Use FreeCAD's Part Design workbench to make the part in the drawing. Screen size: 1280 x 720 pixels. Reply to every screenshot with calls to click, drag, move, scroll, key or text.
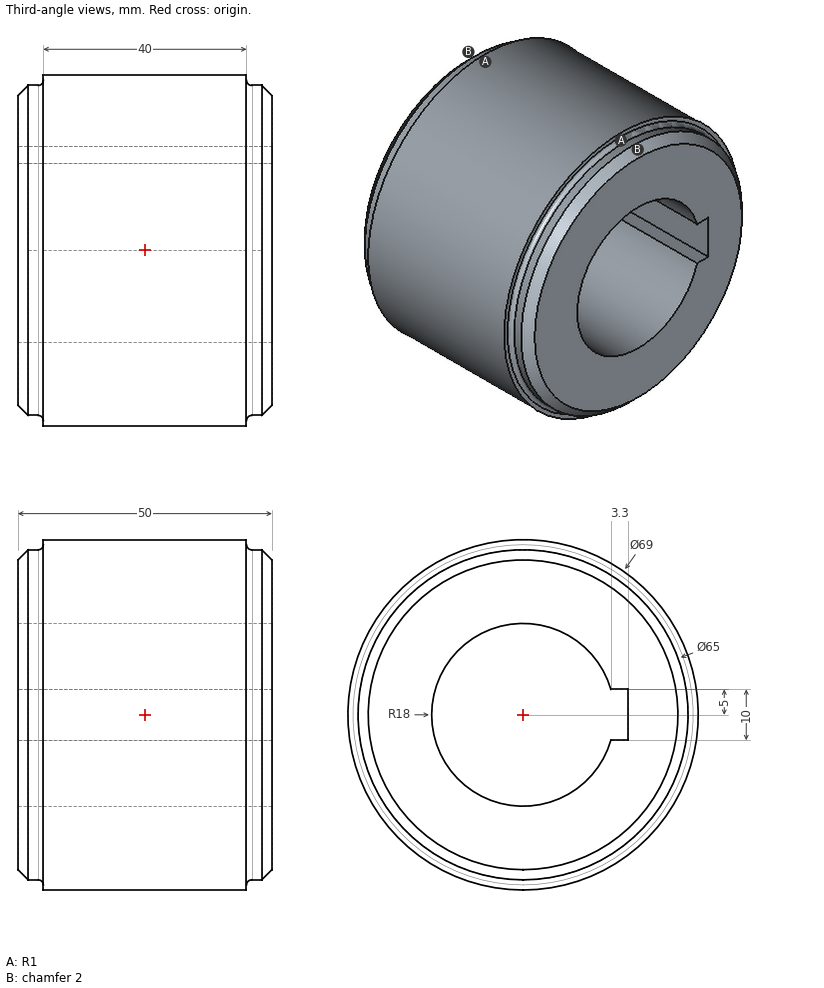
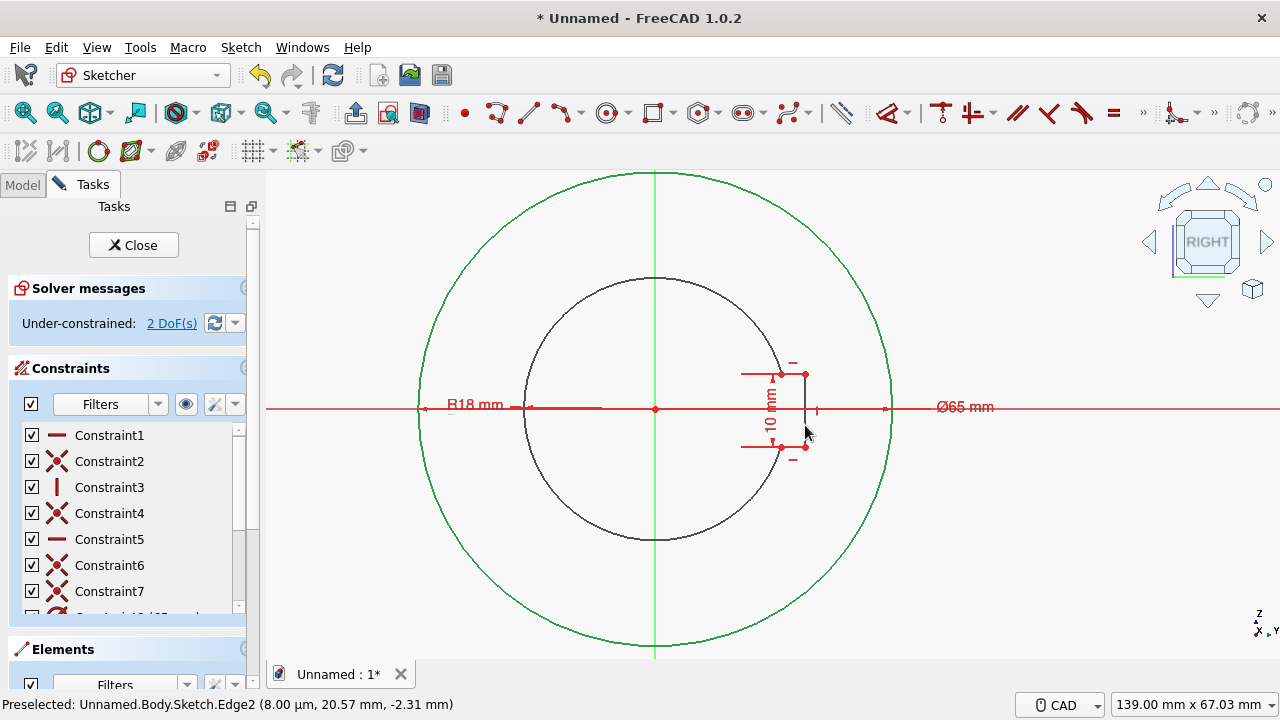
click(782, 374)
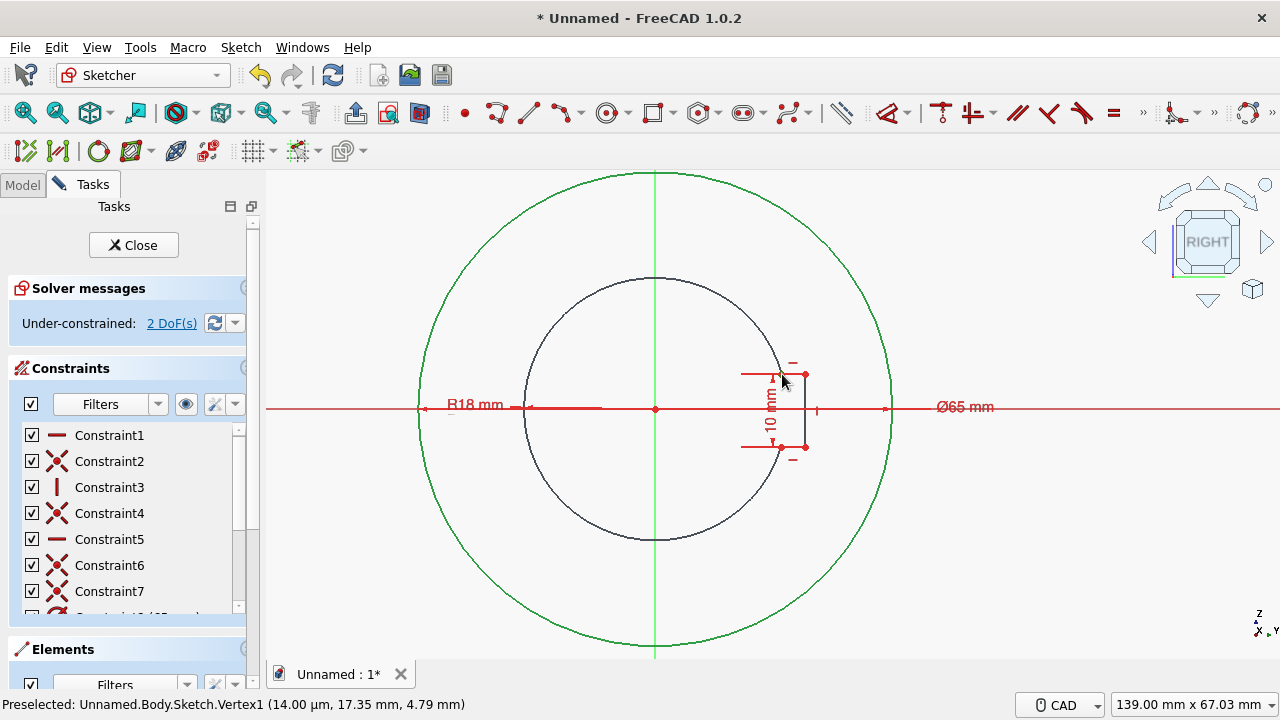
key(i)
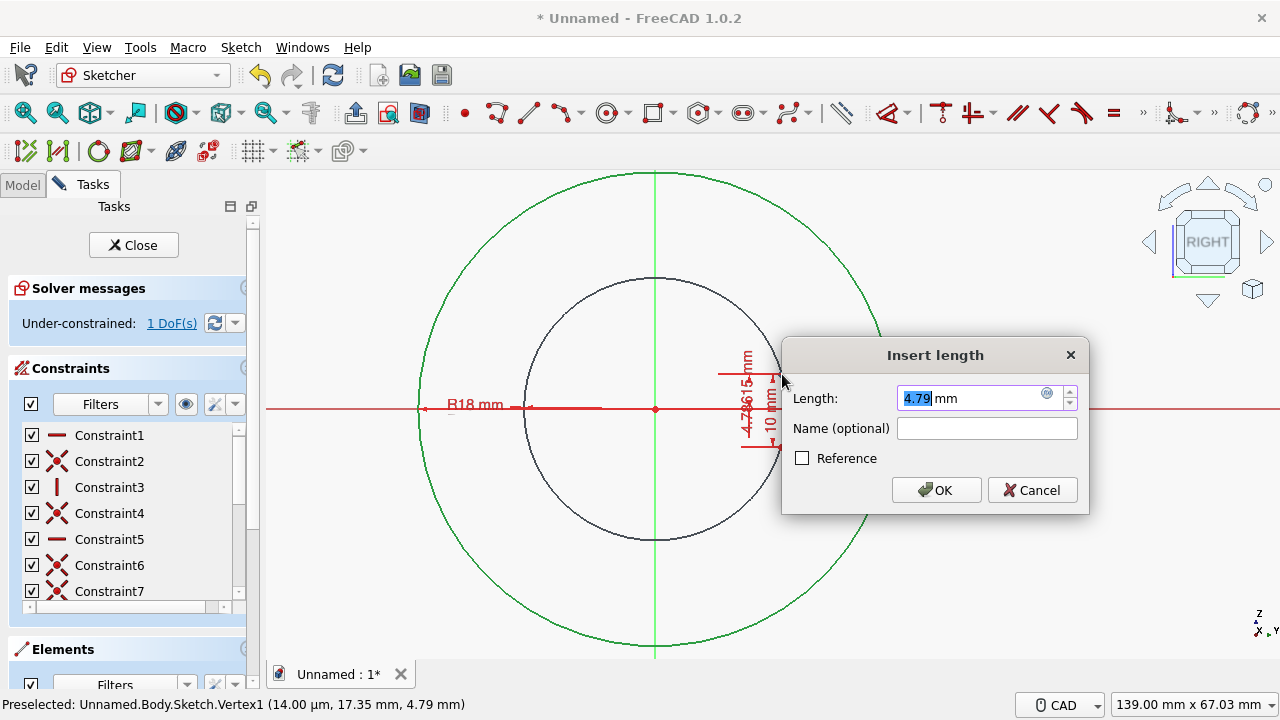
text(5)
key(Return)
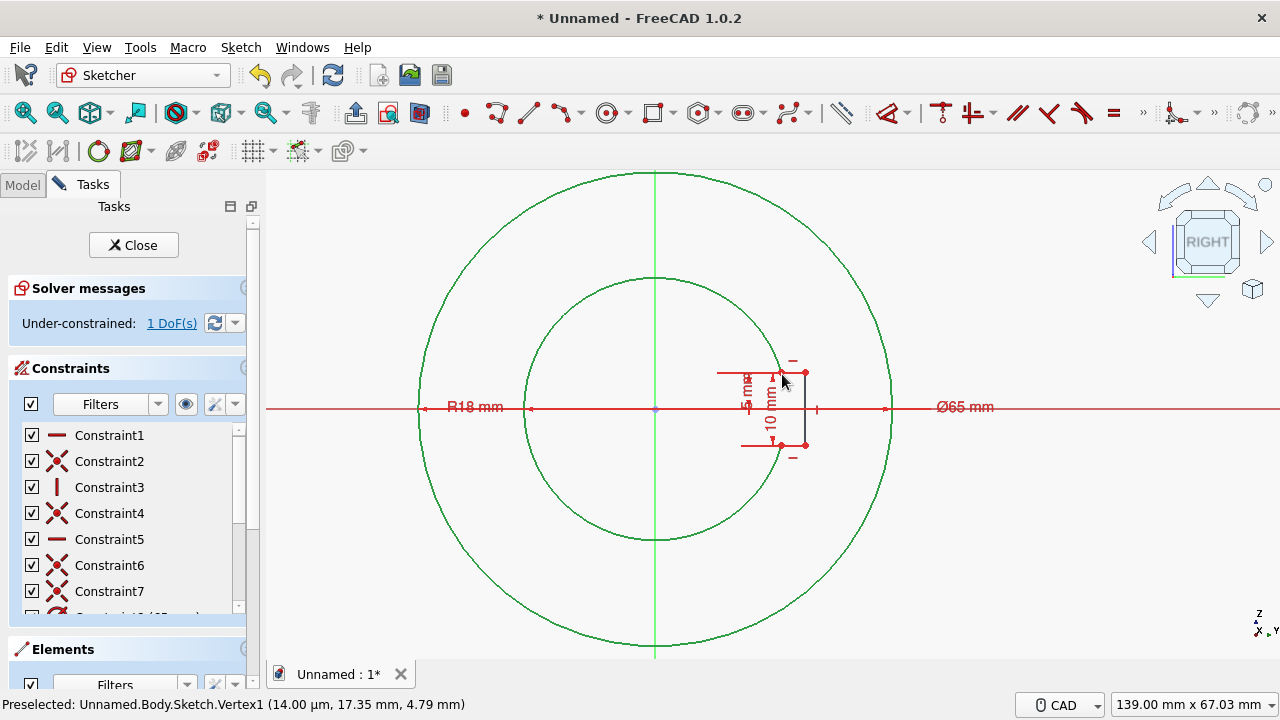
scroll(791, 373, up, 3)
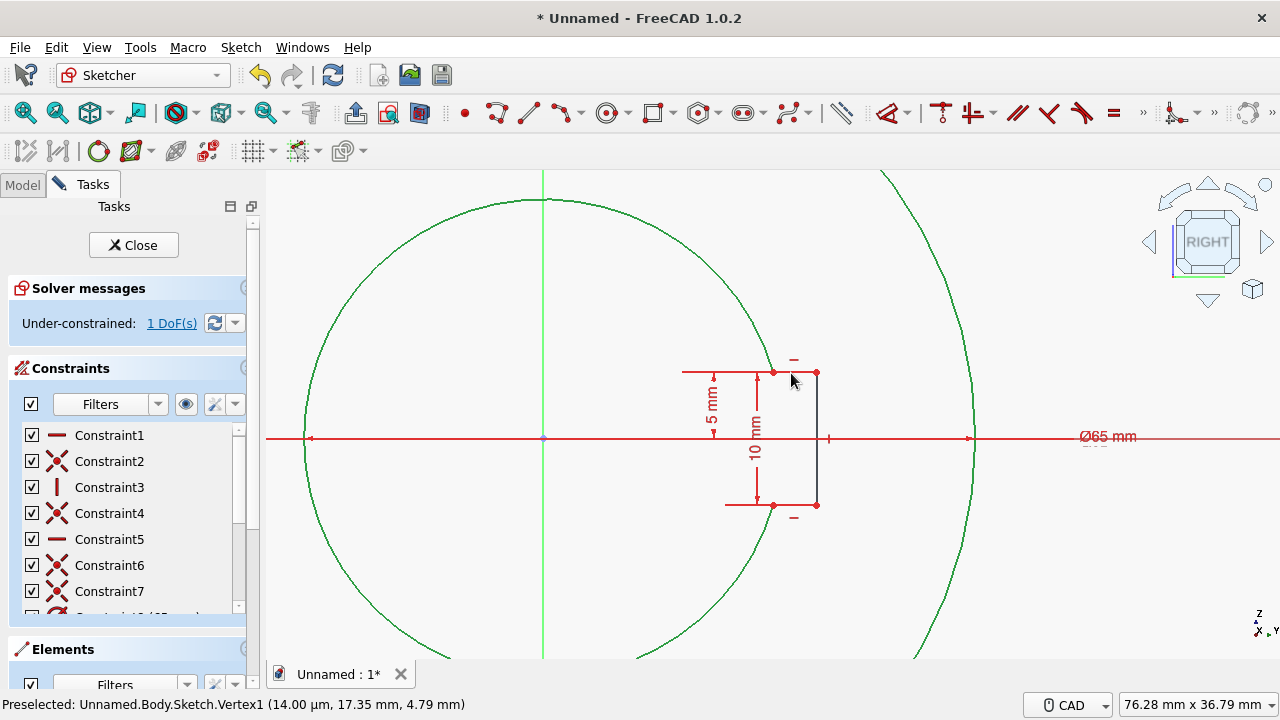
click(791, 372)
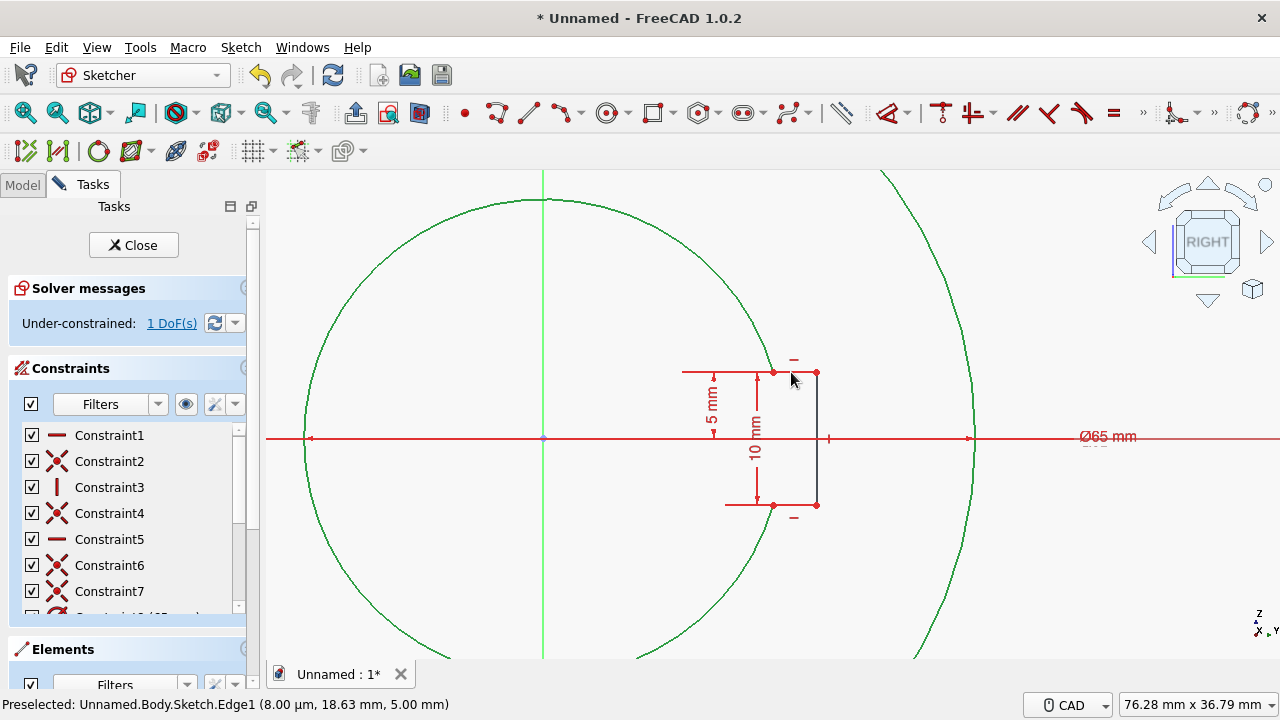
key(l)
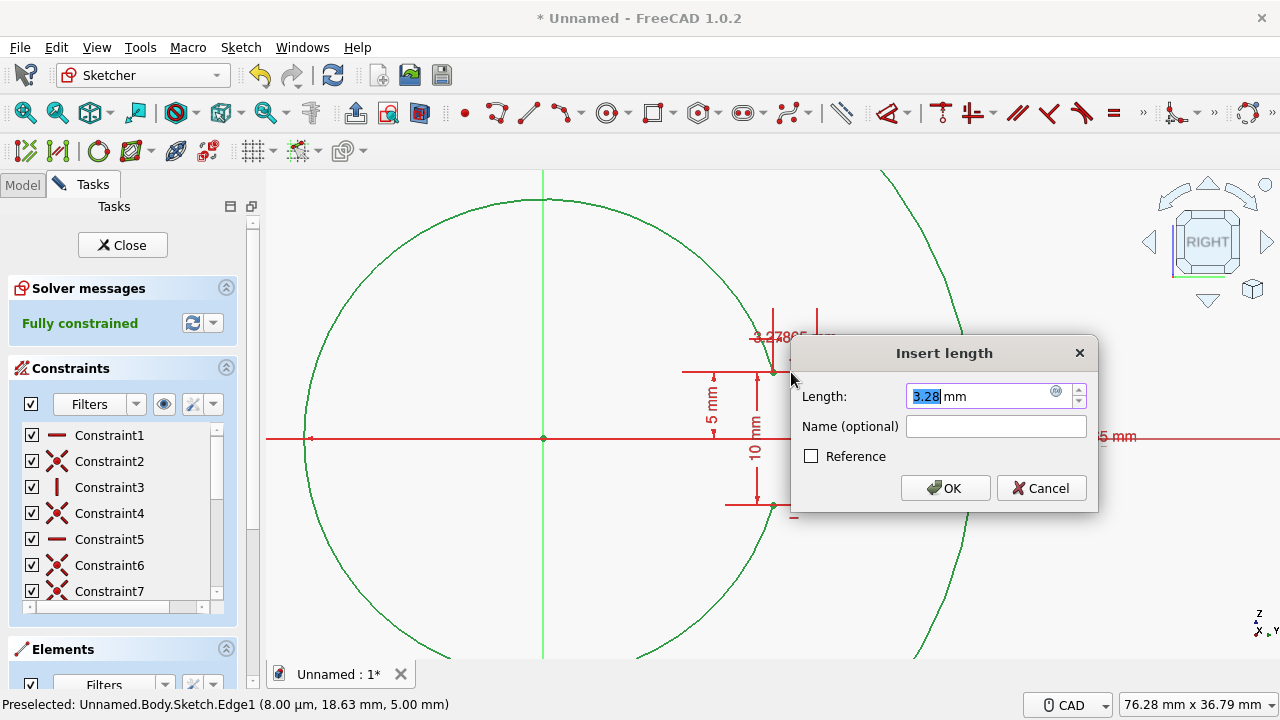
text(3.3)
key(Return)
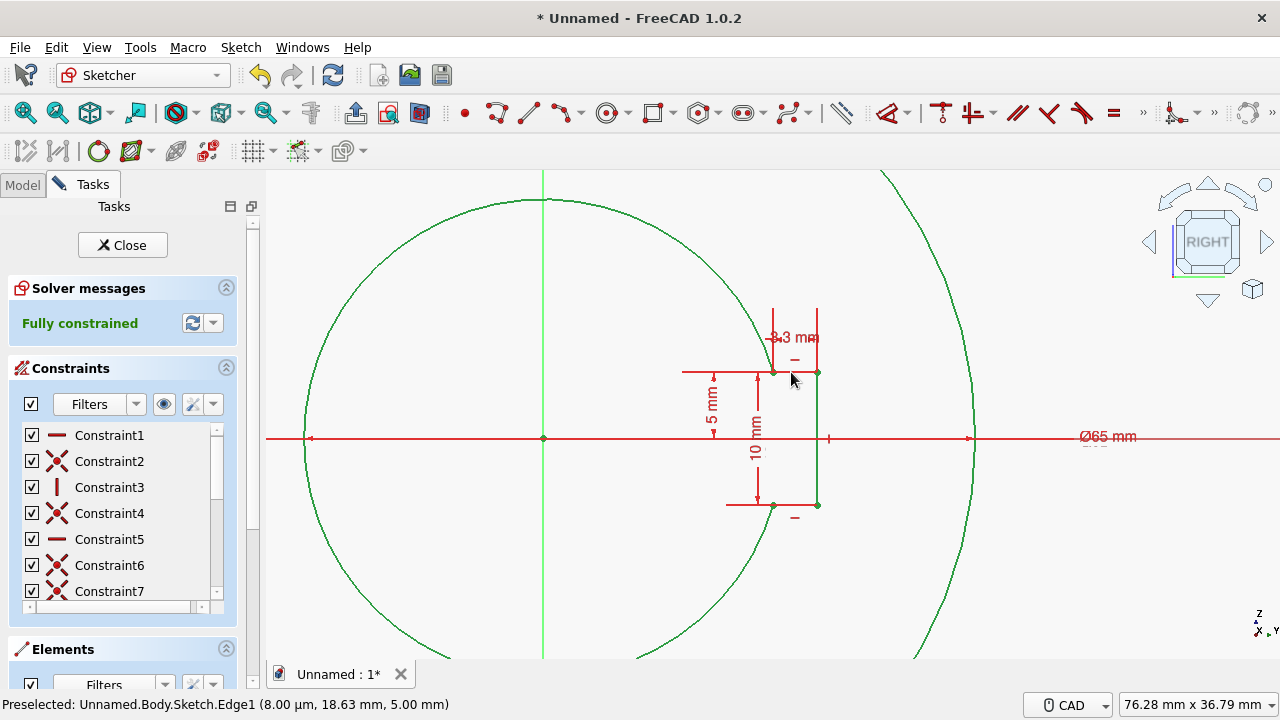
click(123, 245)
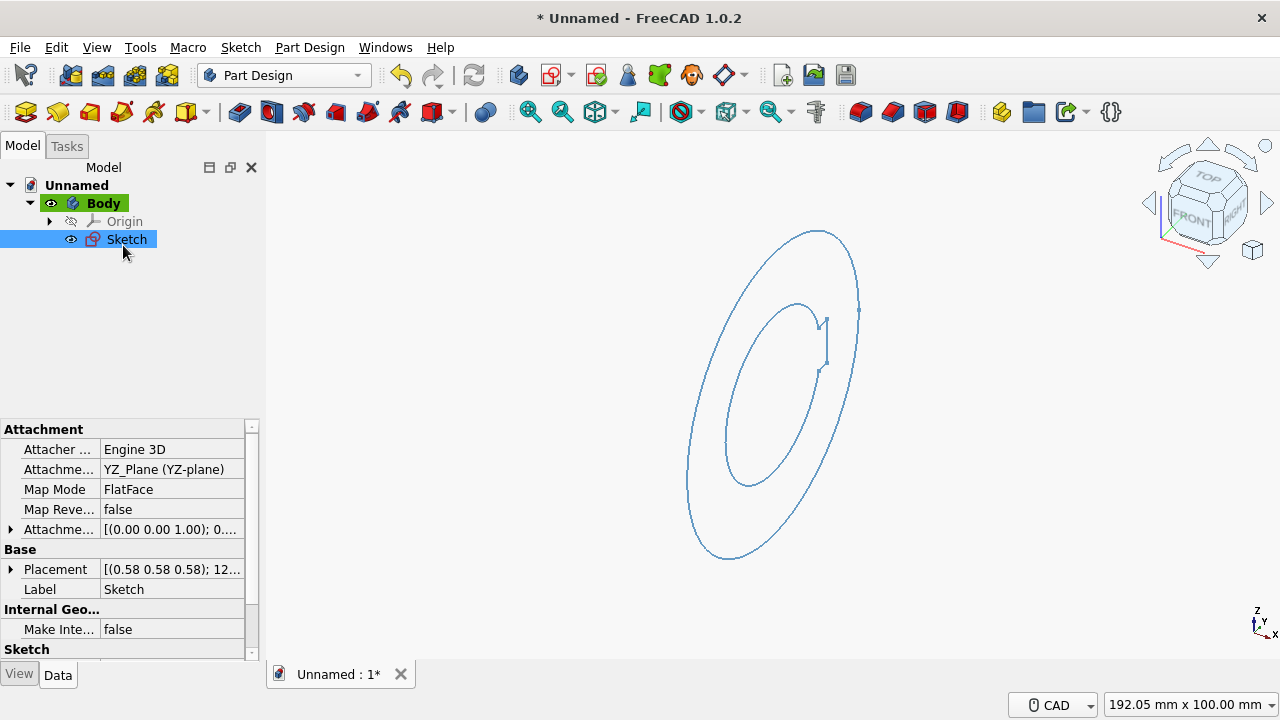
click(26, 112)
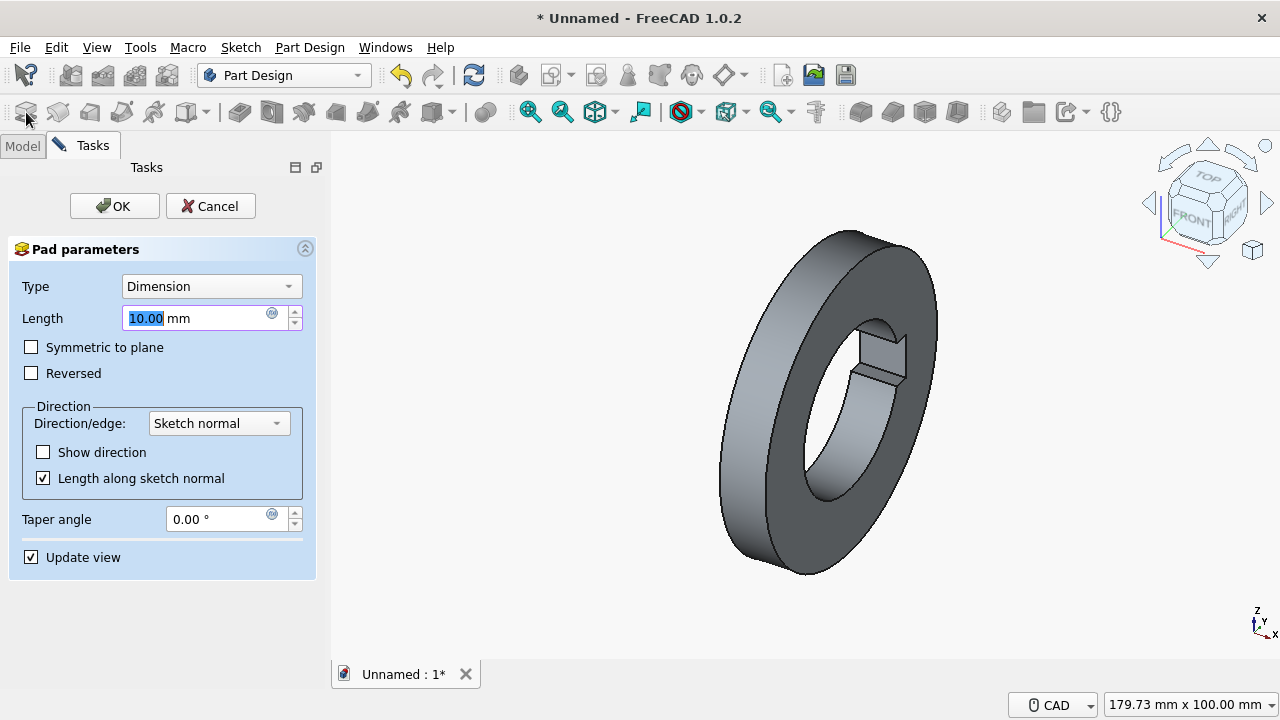
text(50)
key(Tab)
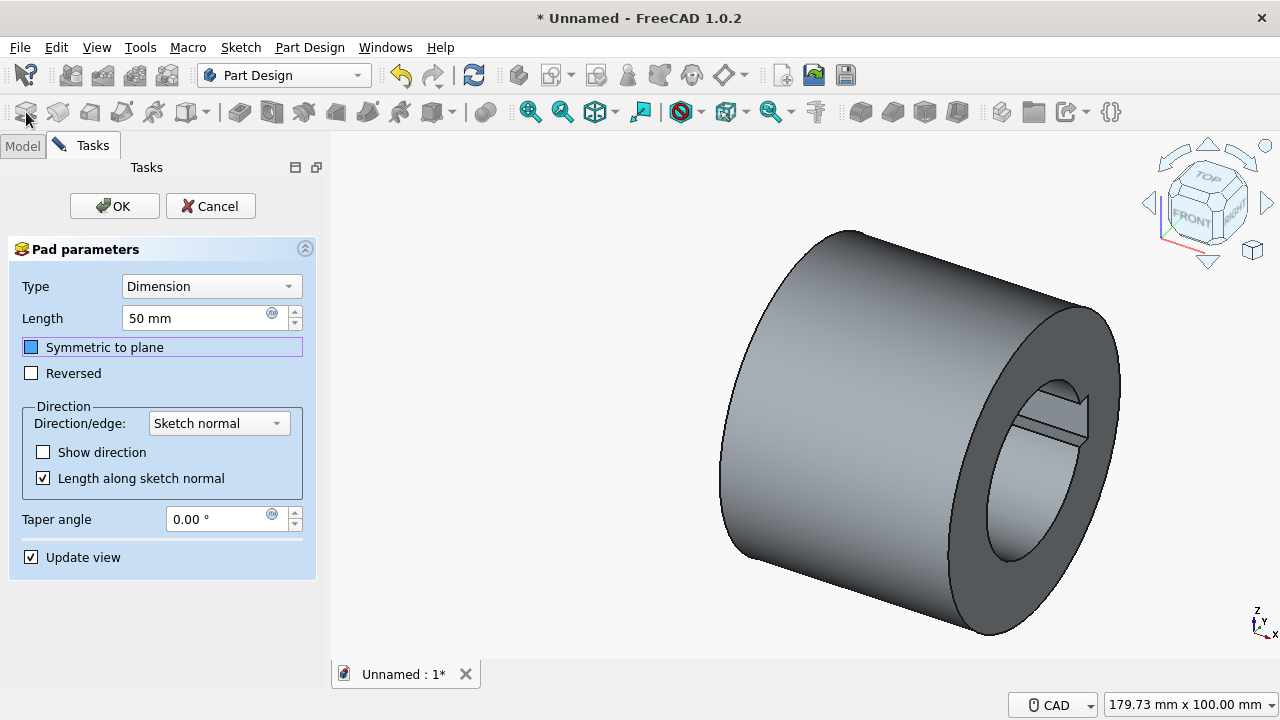
click(30, 347)